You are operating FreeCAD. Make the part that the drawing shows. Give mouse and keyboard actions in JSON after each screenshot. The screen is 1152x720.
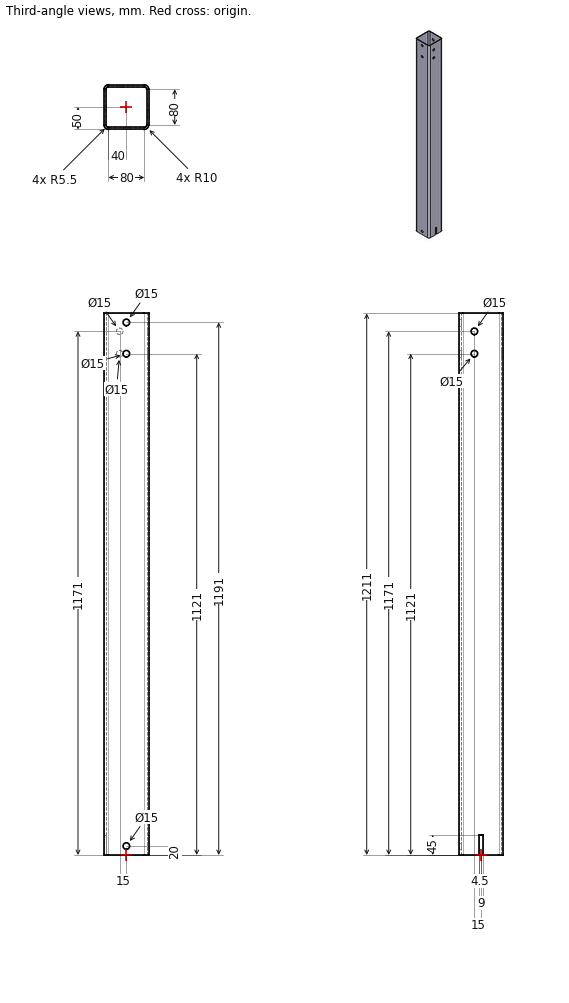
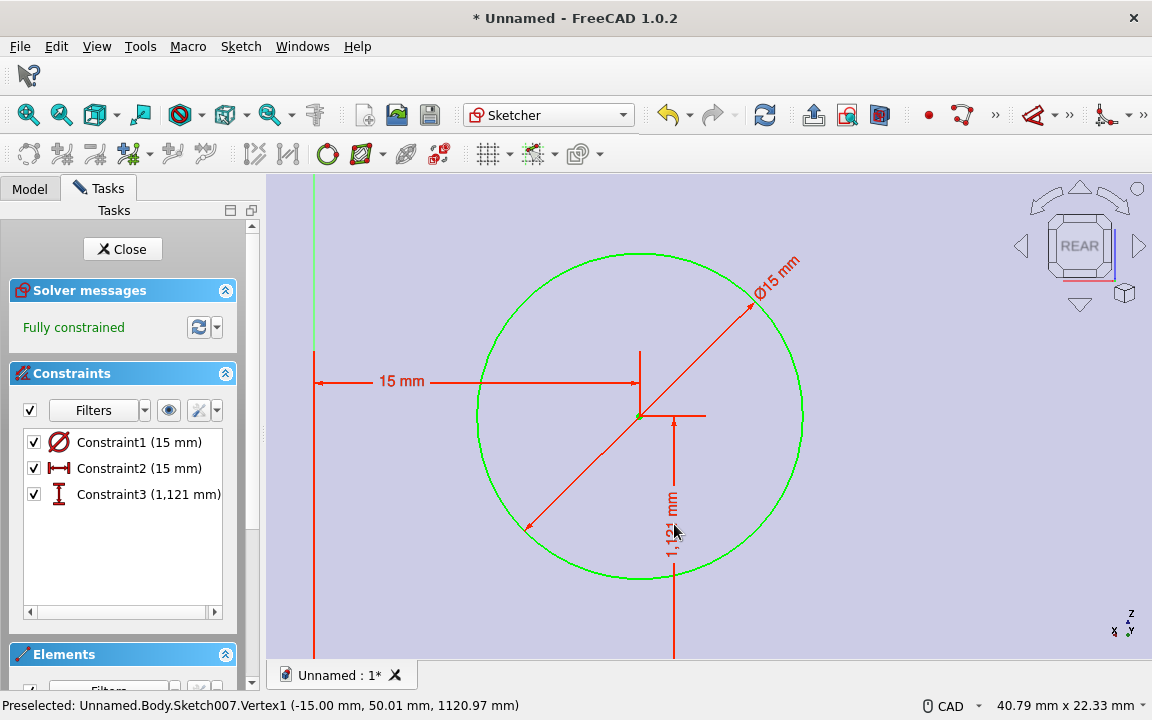
{"action": "left_click", "coordinate": [123, 249]}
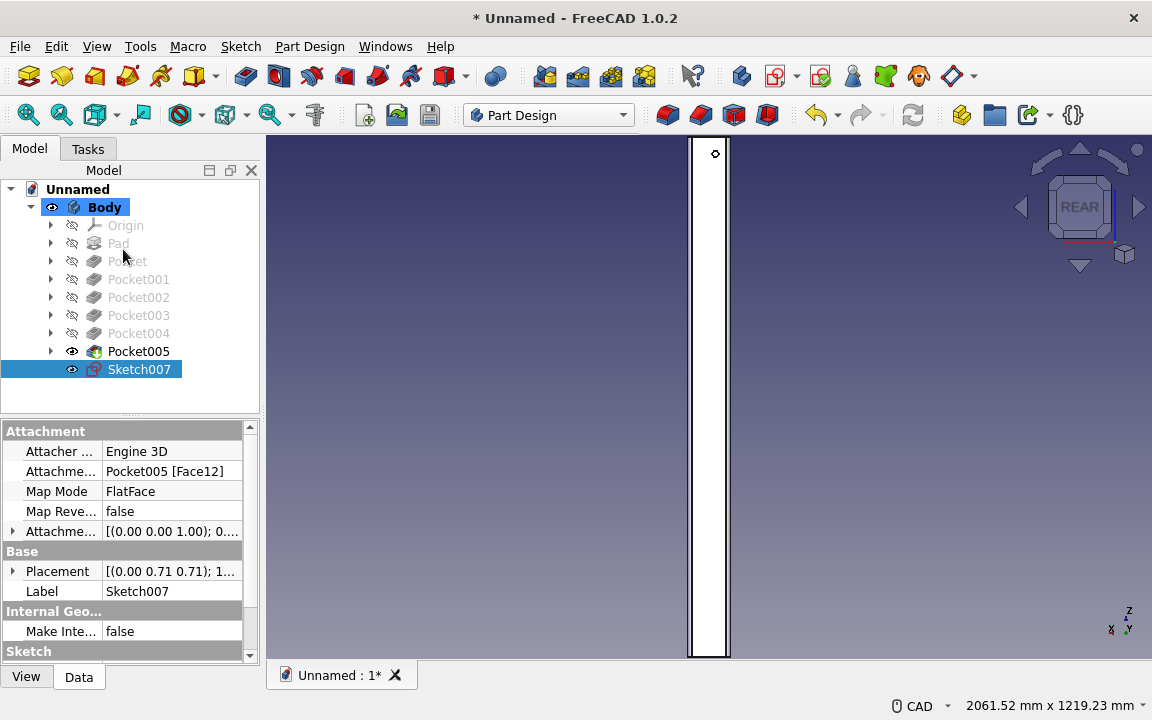
{"action": "left_click", "coordinate": [246, 76]}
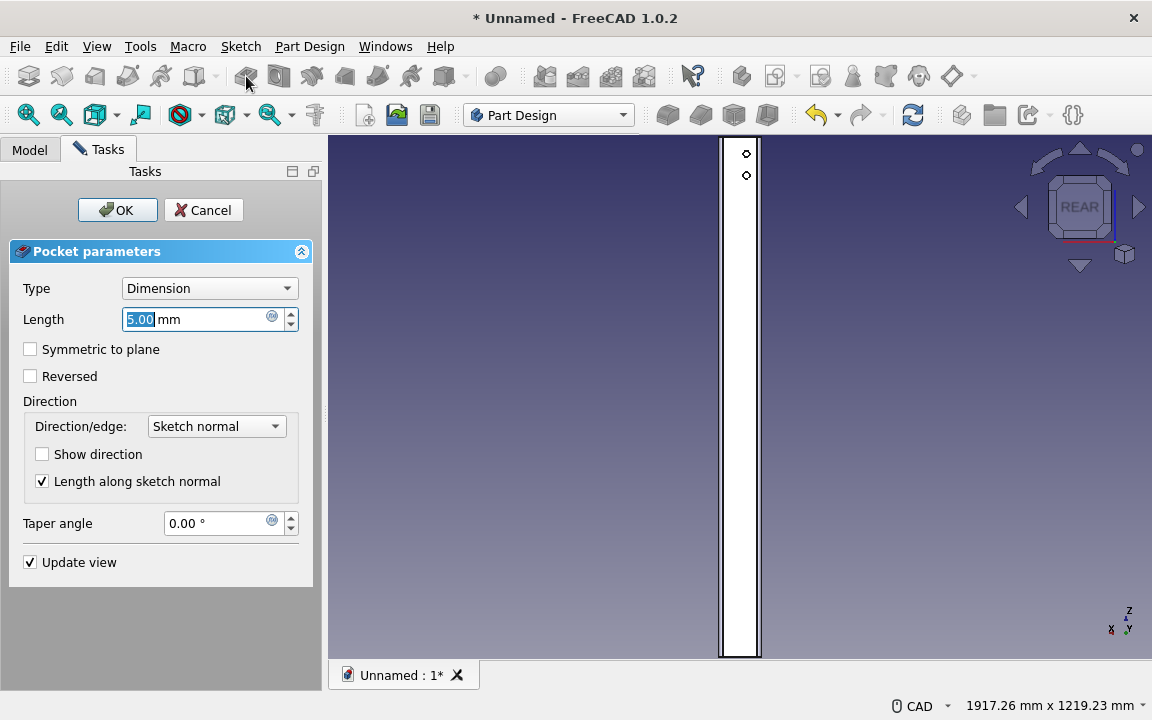
{"action": "left_click", "coordinate": [210, 288]}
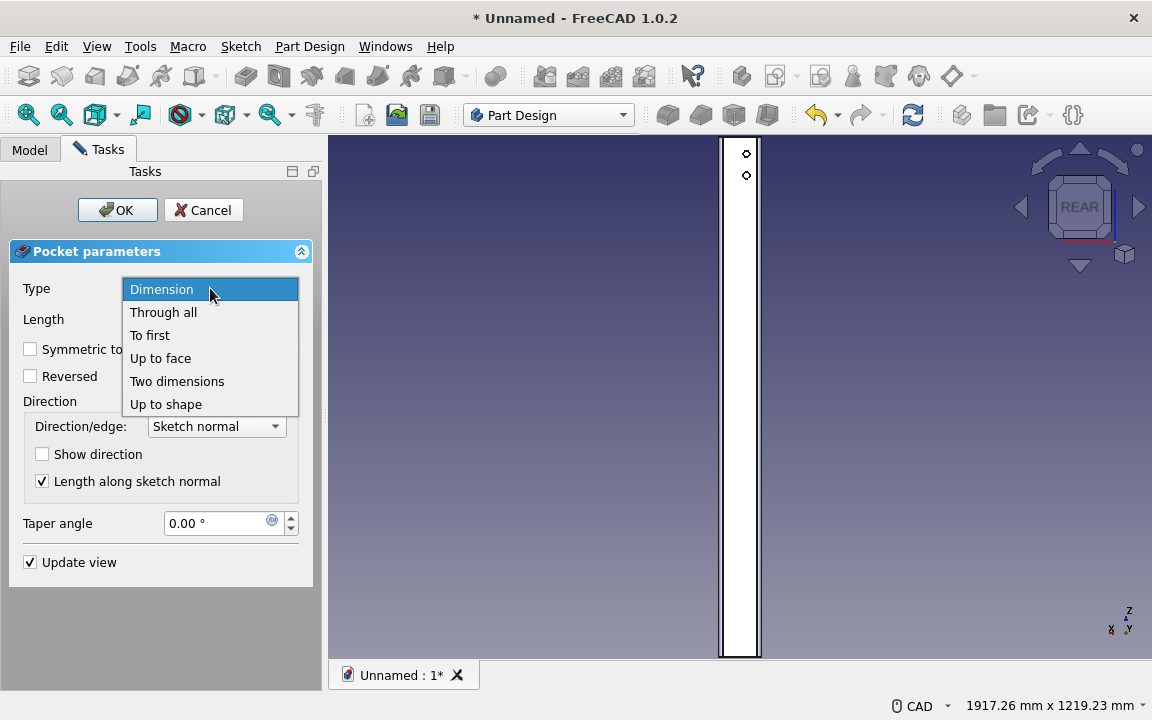
{"action": "left_click", "coordinate": [208, 336]}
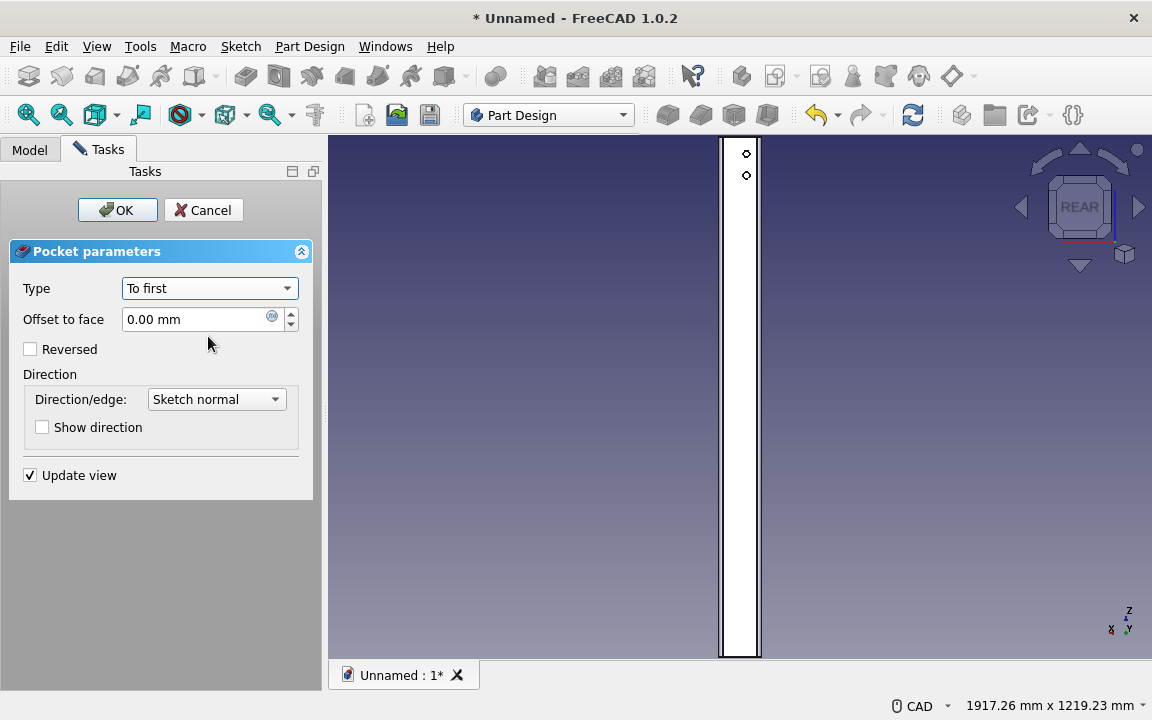
{"action": "left_click", "coordinate": [118, 210]}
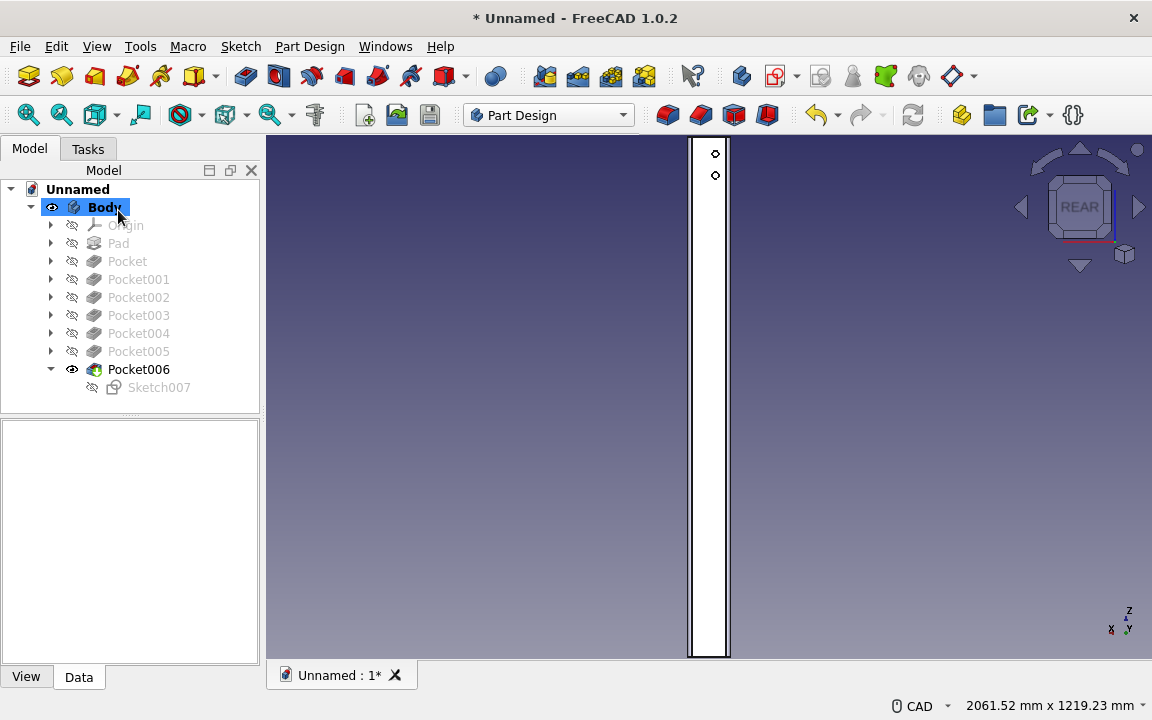
{"action": "key", "text": "0"}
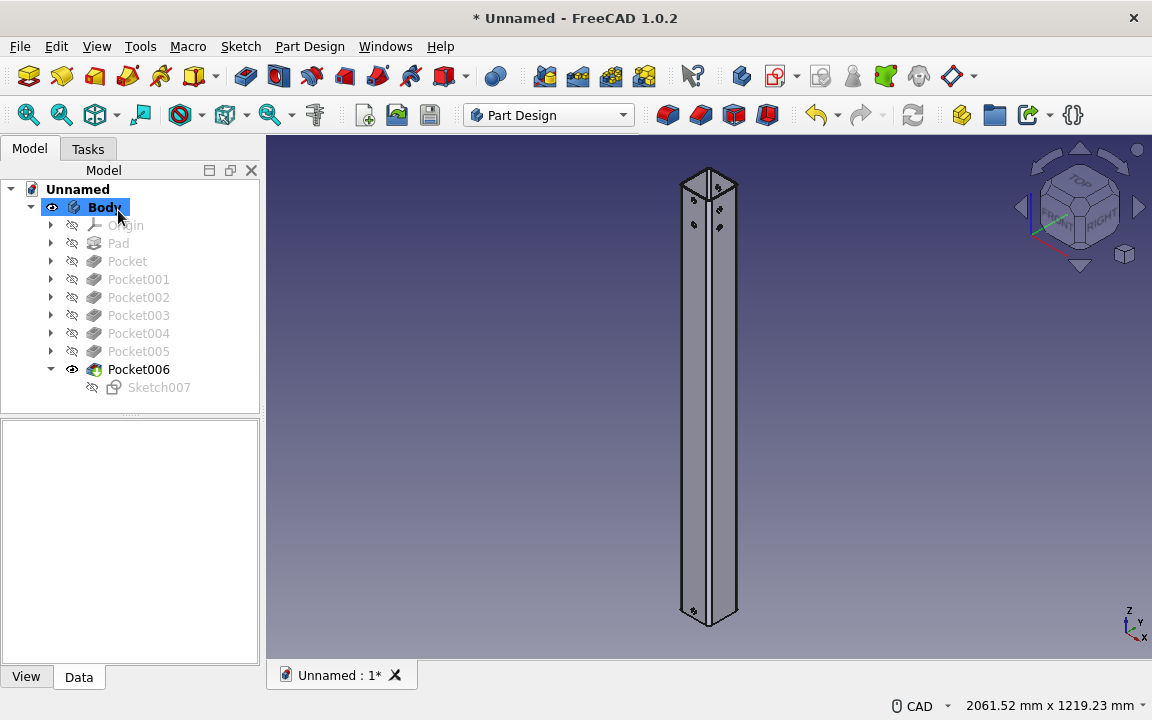
{"action": "left_click", "coordinate": [724, 283]}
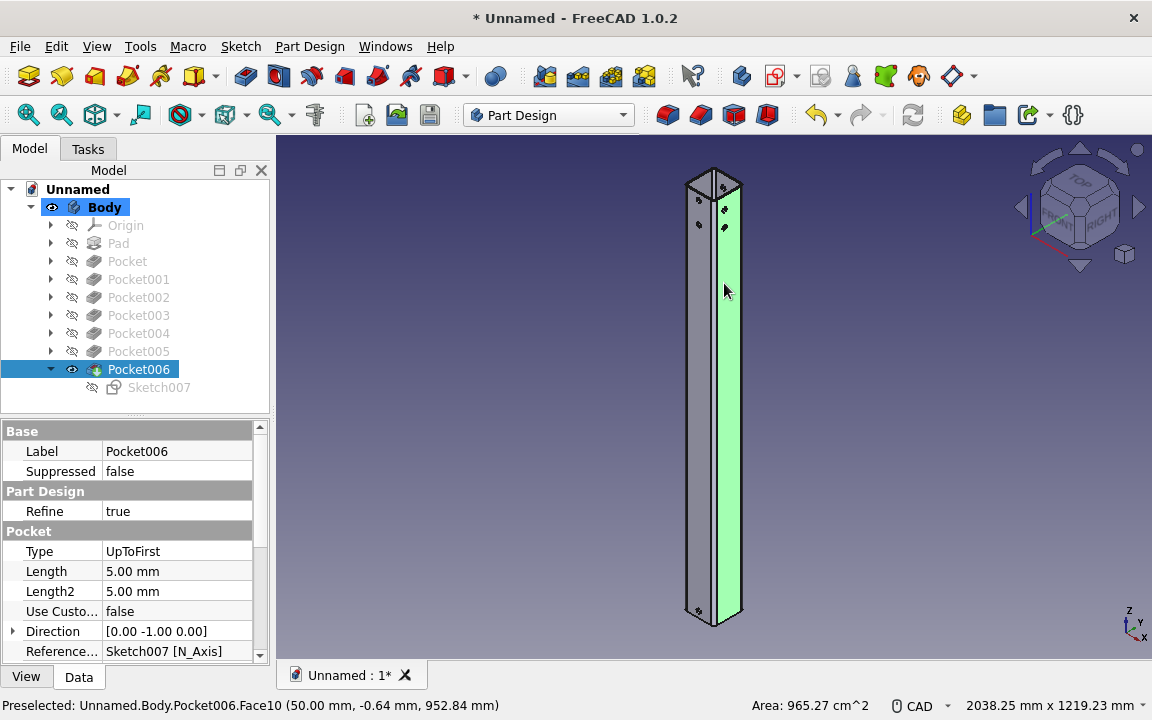
{"action": "left_click", "coordinate": [774, 76]}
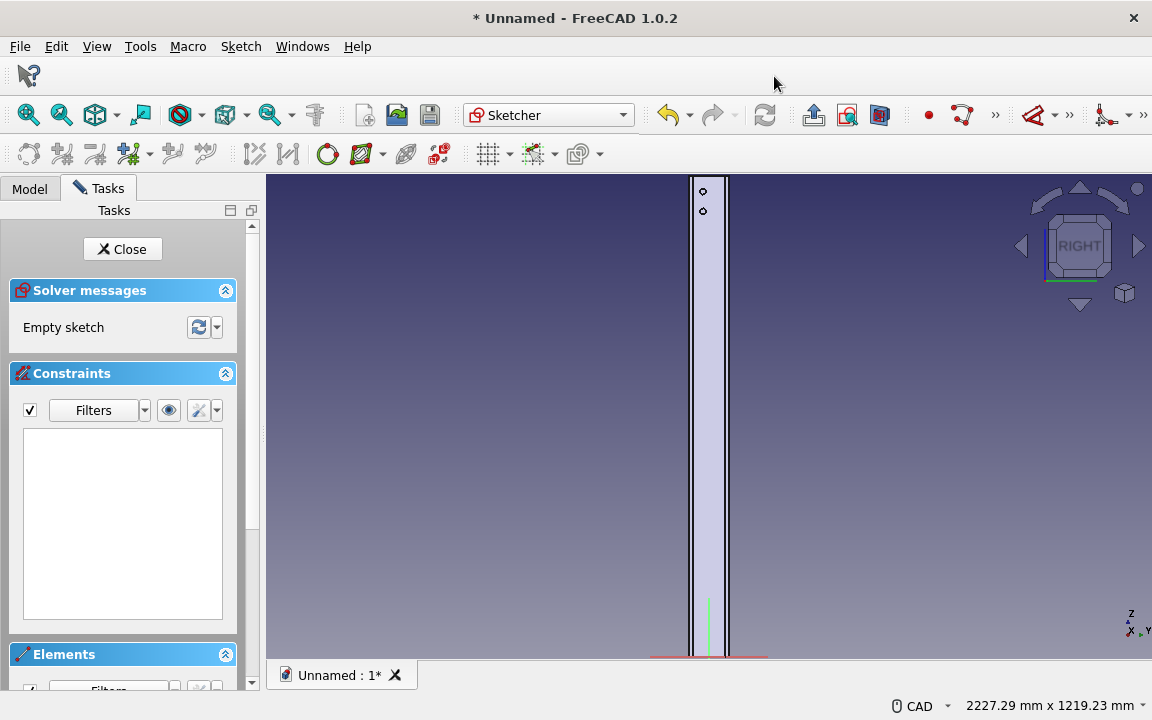
{"action": "scroll", "coordinate": [640, 416], "scroll_direction": "down", "scroll_amount": 5}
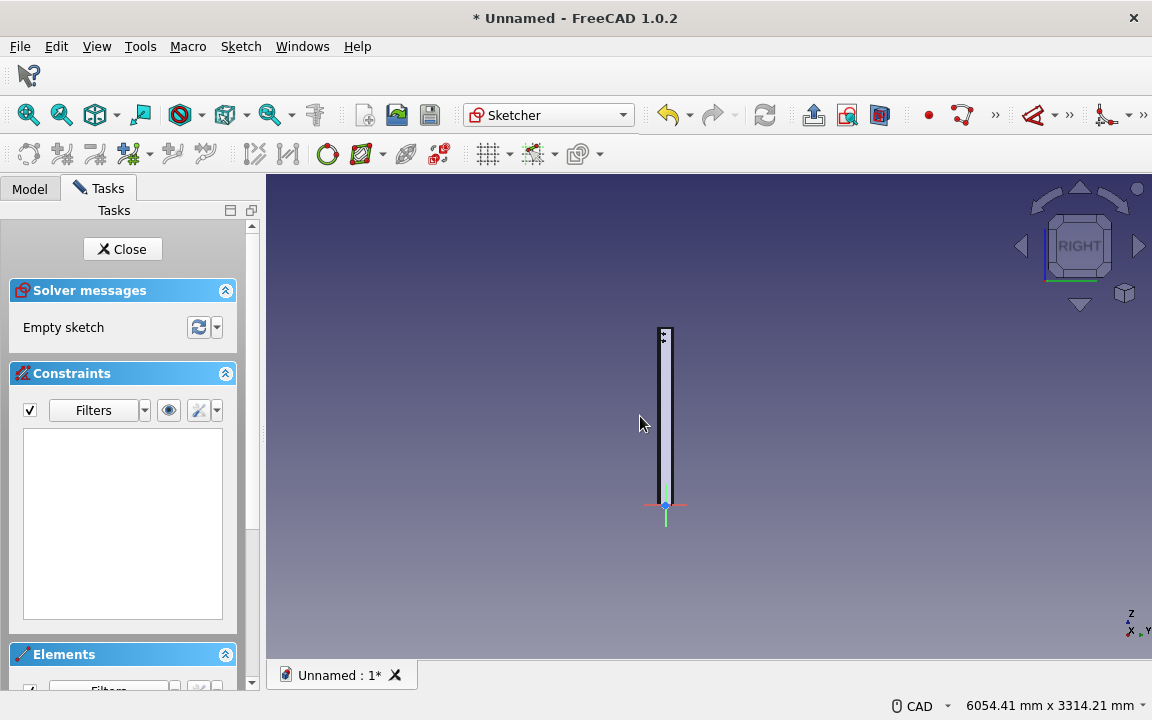
{"action": "scroll", "coordinate": [667, 506], "scroll_direction": "up", "scroll_amount": 15}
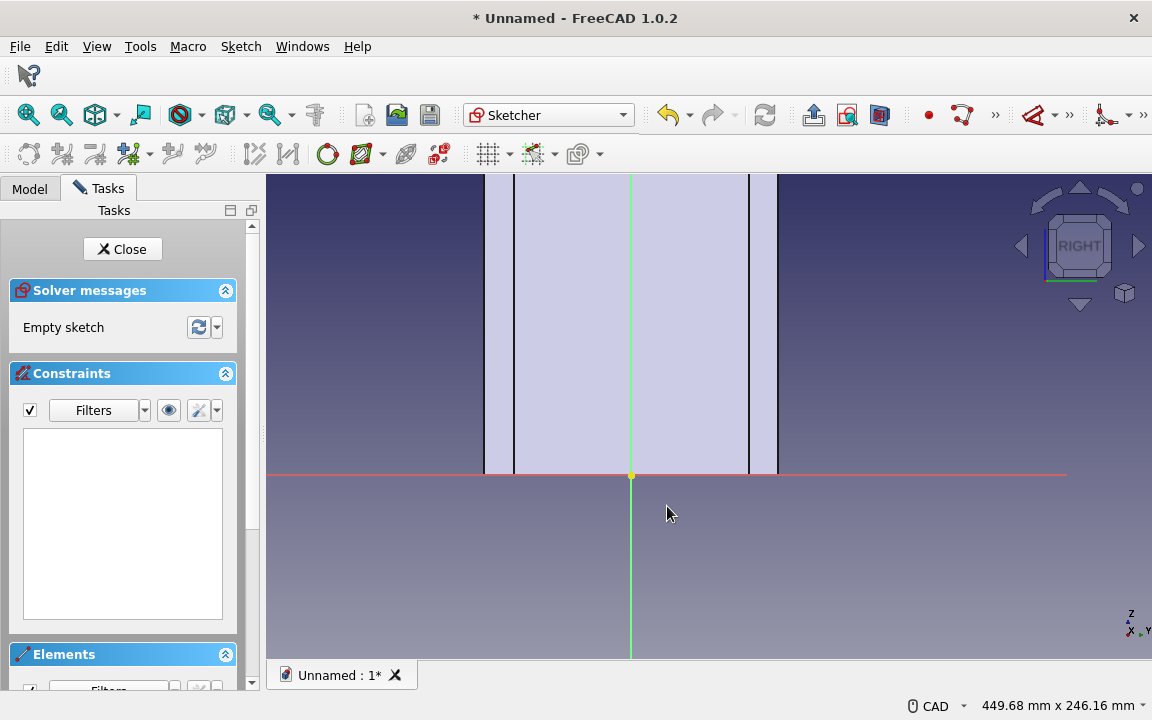
{"action": "scroll", "coordinate": [624, 403], "scroll_direction": "up", "scroll_amount": 4}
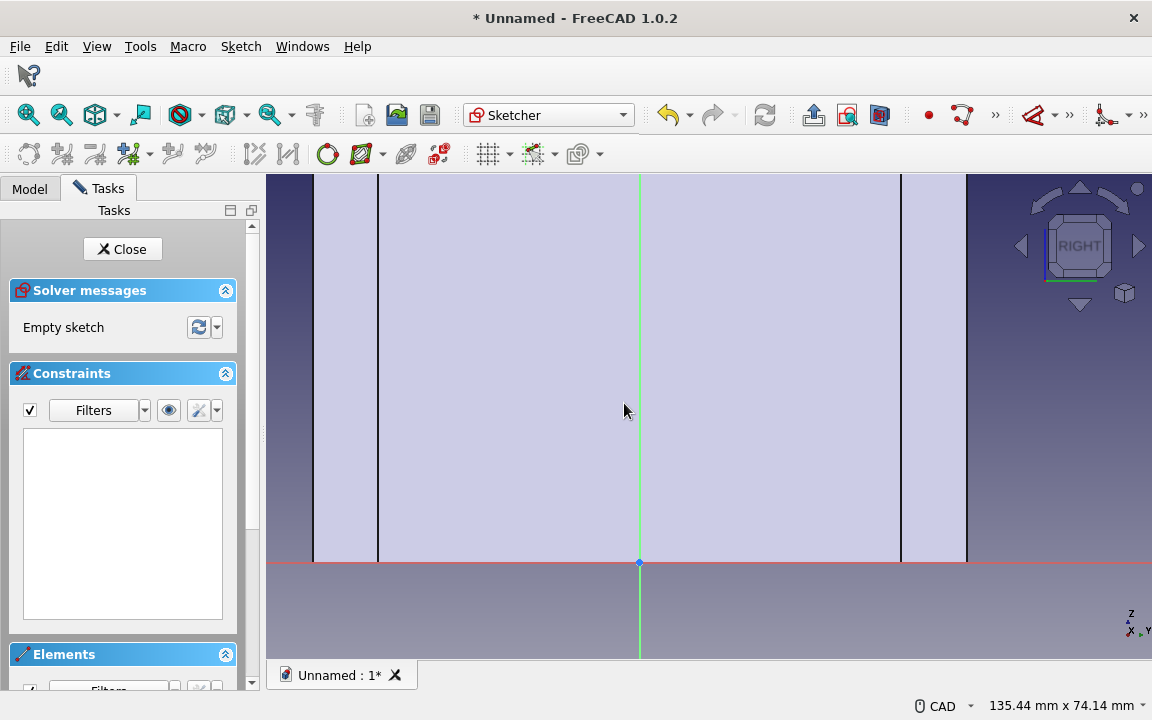
{"action": "key", "text": "g r"}